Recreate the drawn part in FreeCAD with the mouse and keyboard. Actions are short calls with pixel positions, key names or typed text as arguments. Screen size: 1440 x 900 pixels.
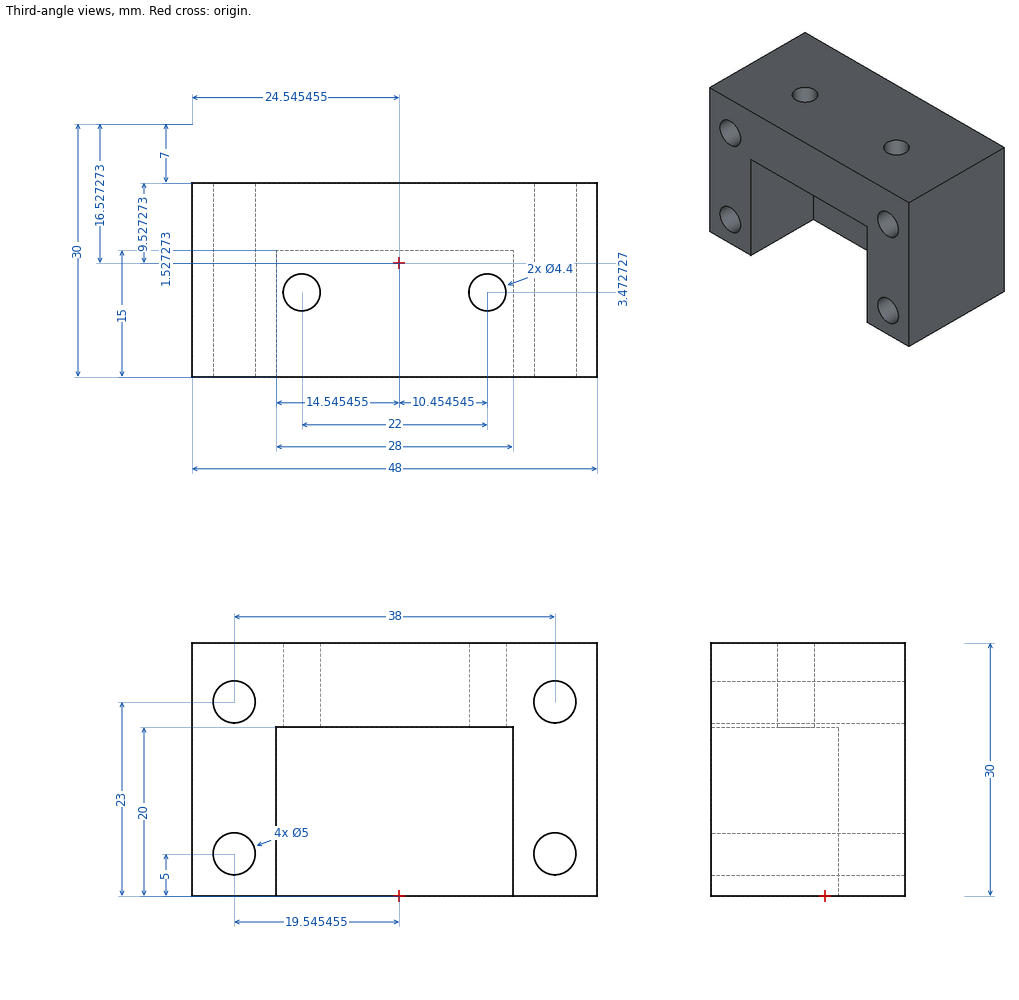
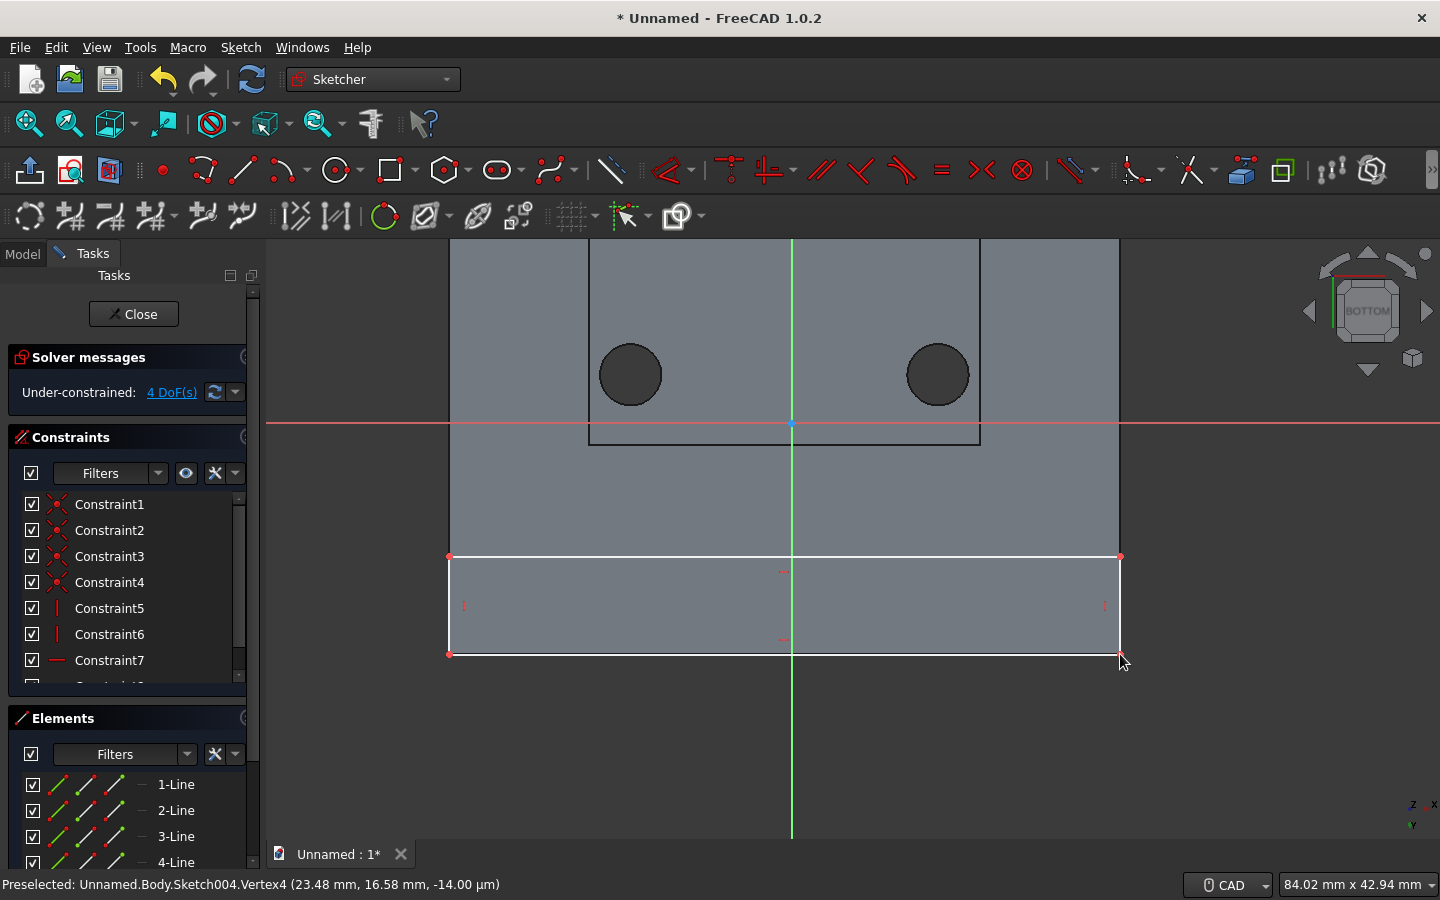
click(666, 170)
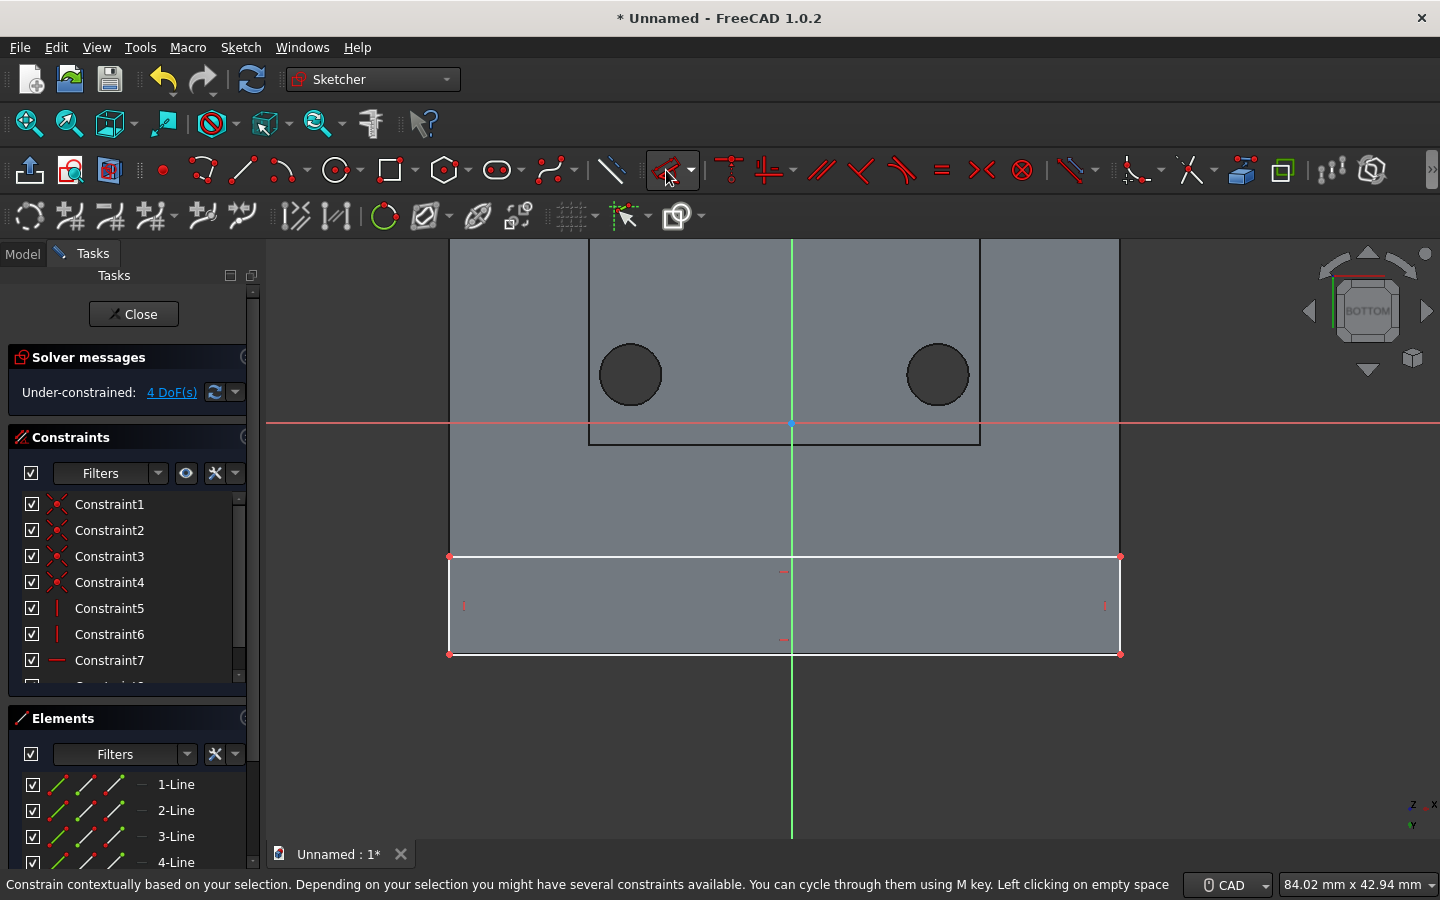
click(449, 586)
click(415, 606)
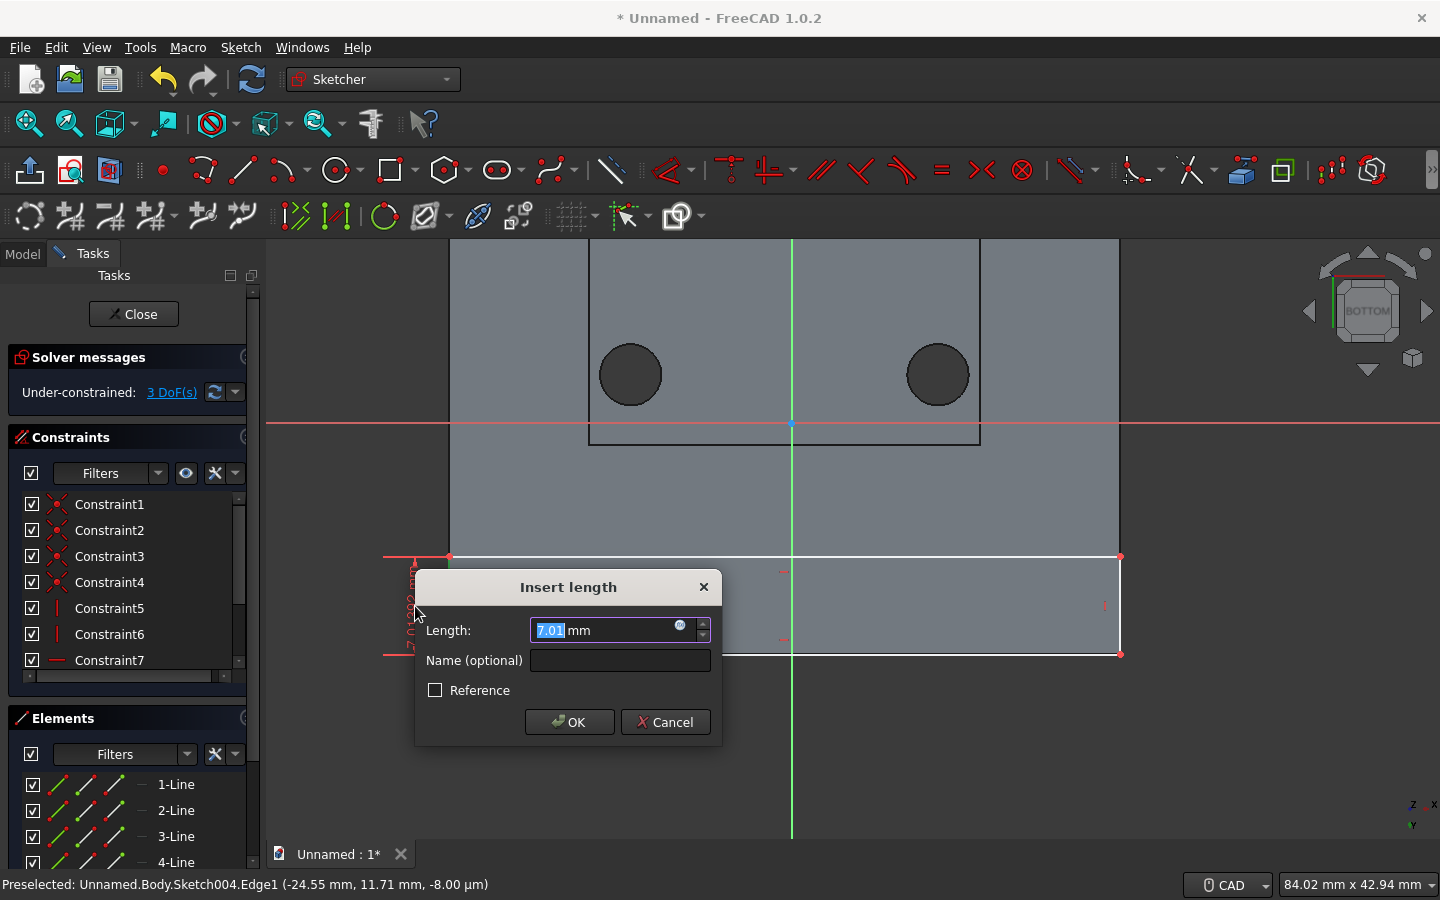
text(7)
key(Return)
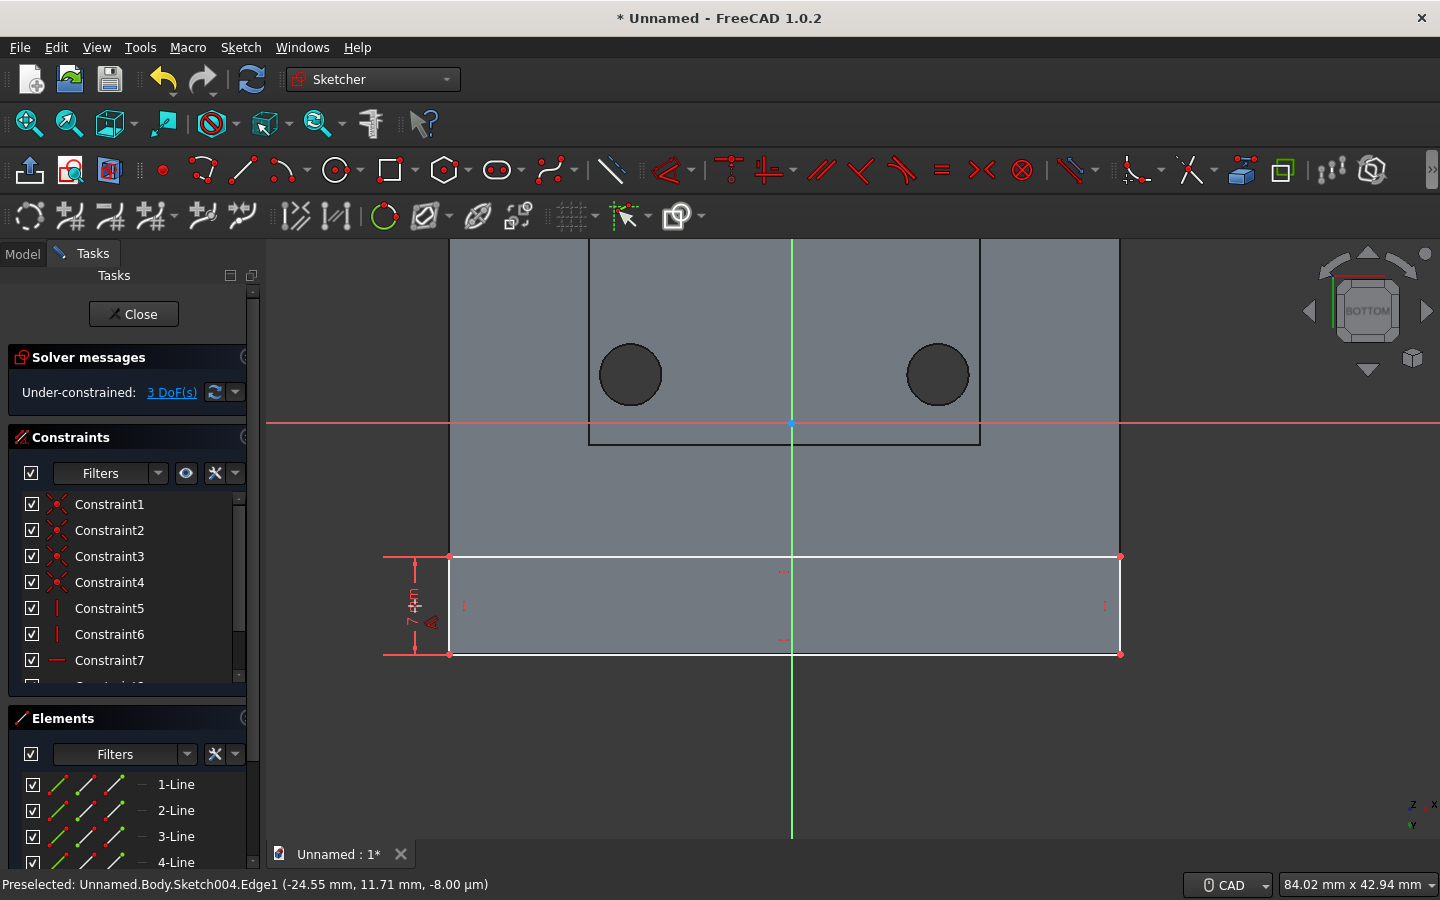
click(650, 655)
click(630, 689)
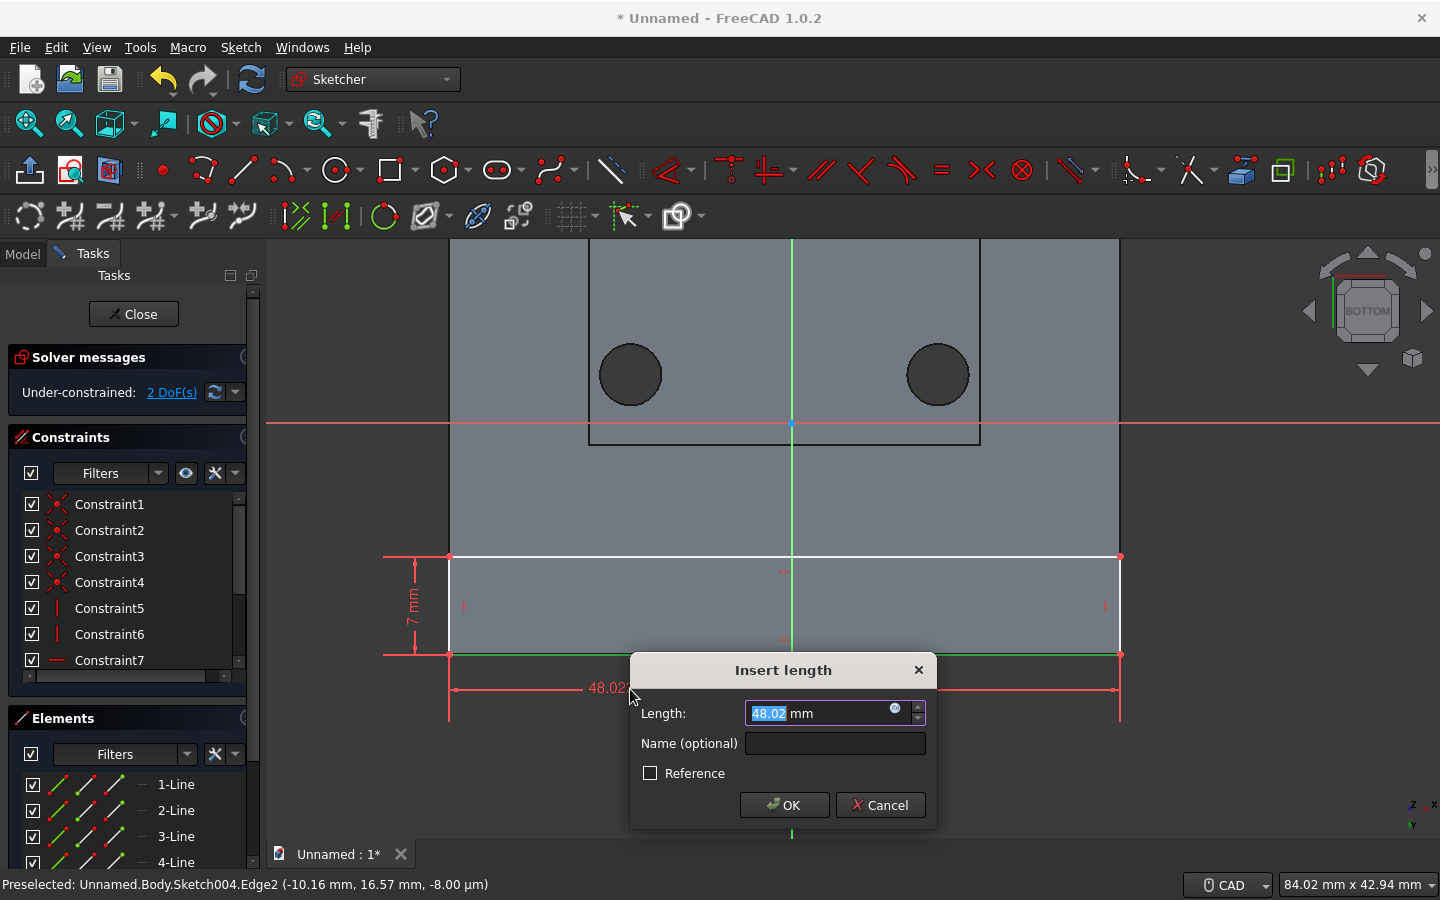
text(48)
key(Return)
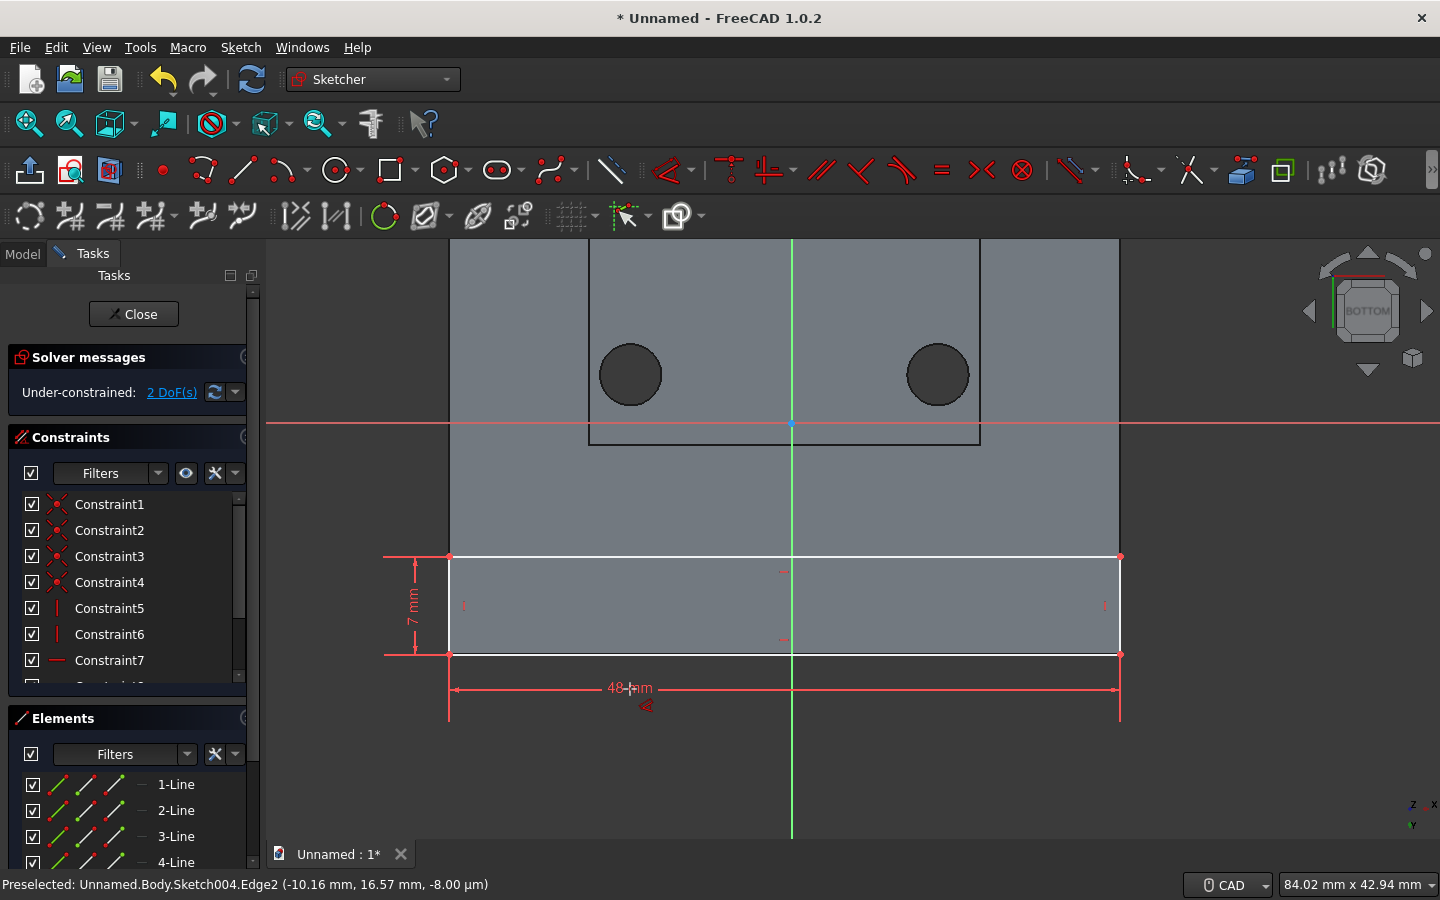
click(449, 557)
click(415, 490)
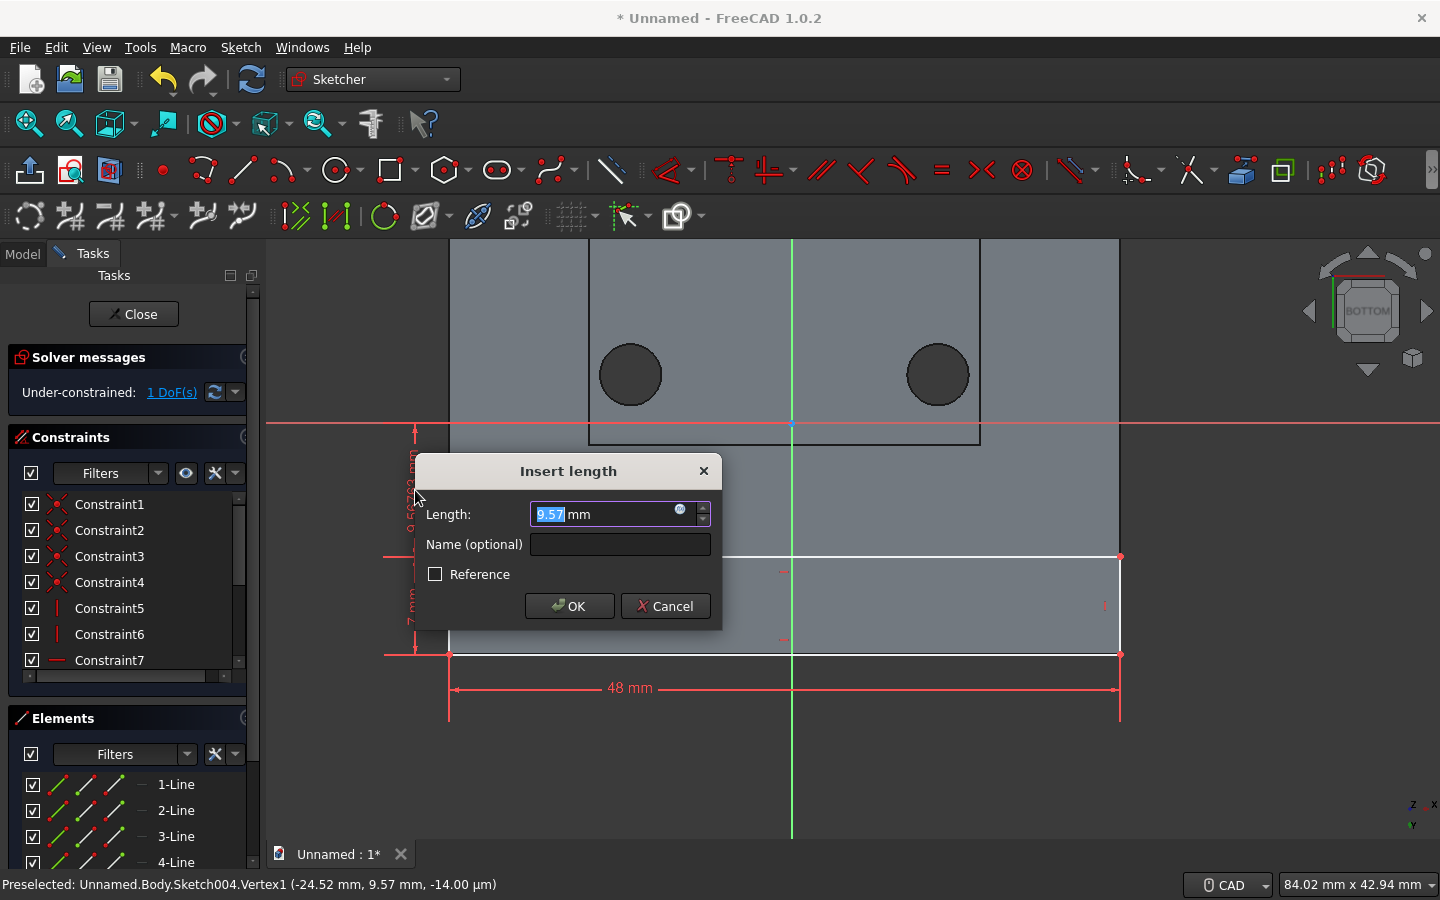
text(9.527273)
key(Return)